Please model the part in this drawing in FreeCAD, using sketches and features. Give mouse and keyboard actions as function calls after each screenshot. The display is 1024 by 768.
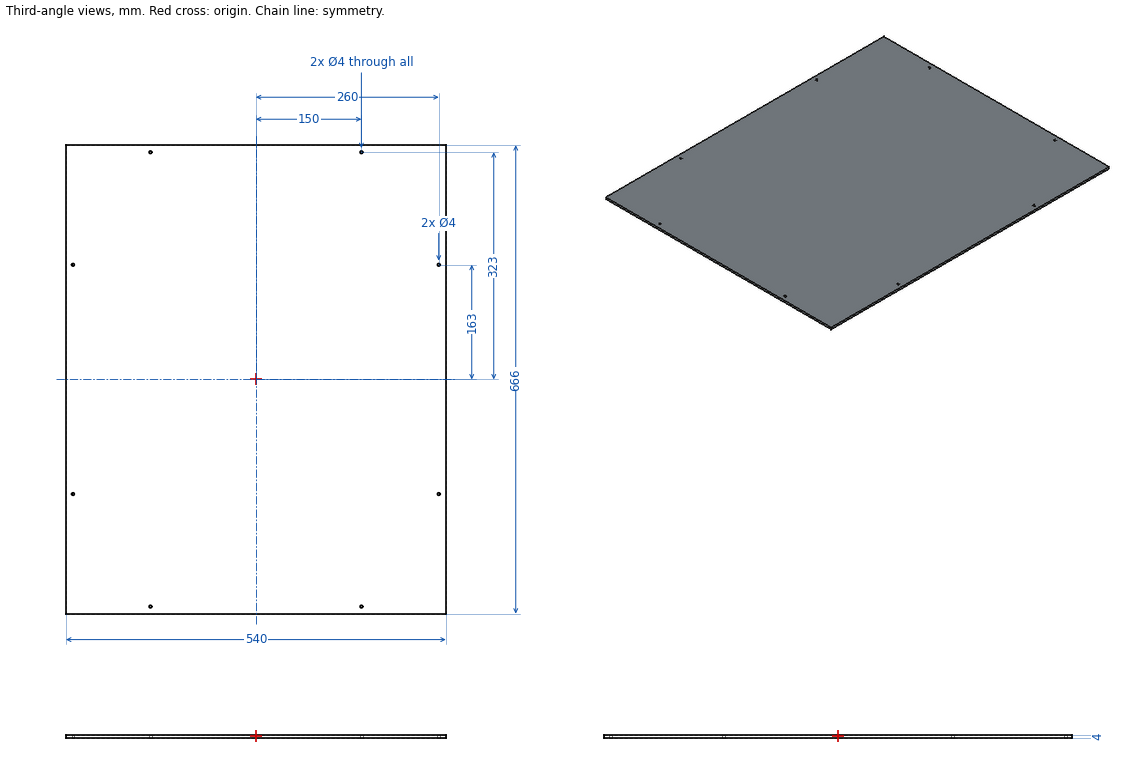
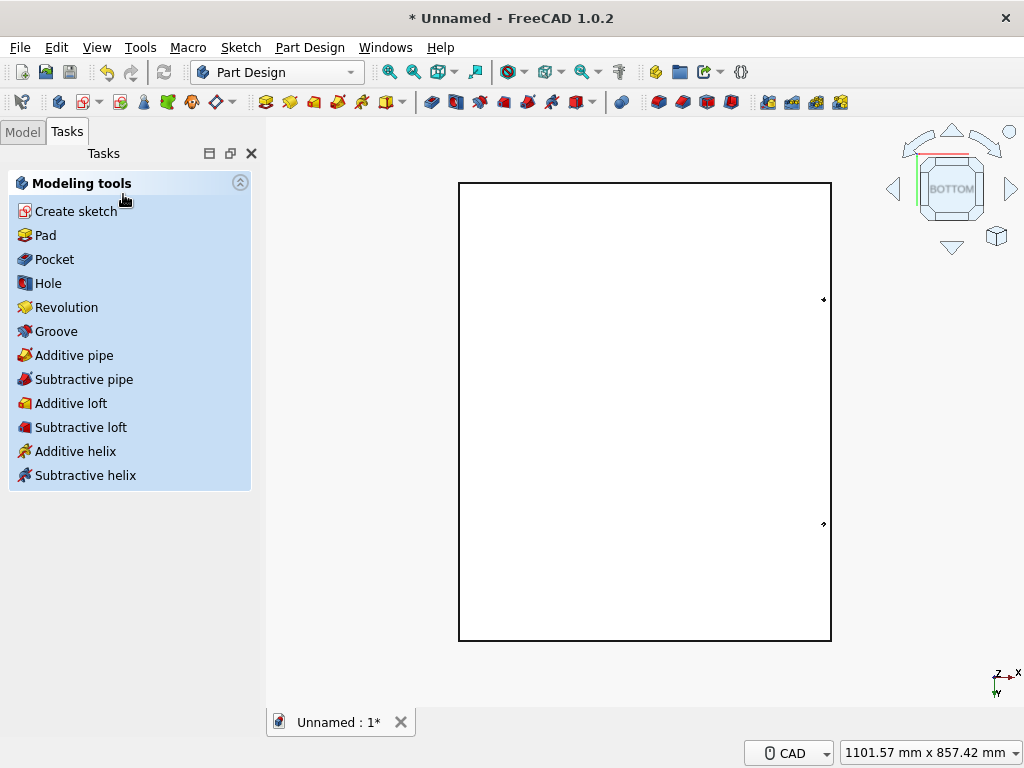
click(456, 102)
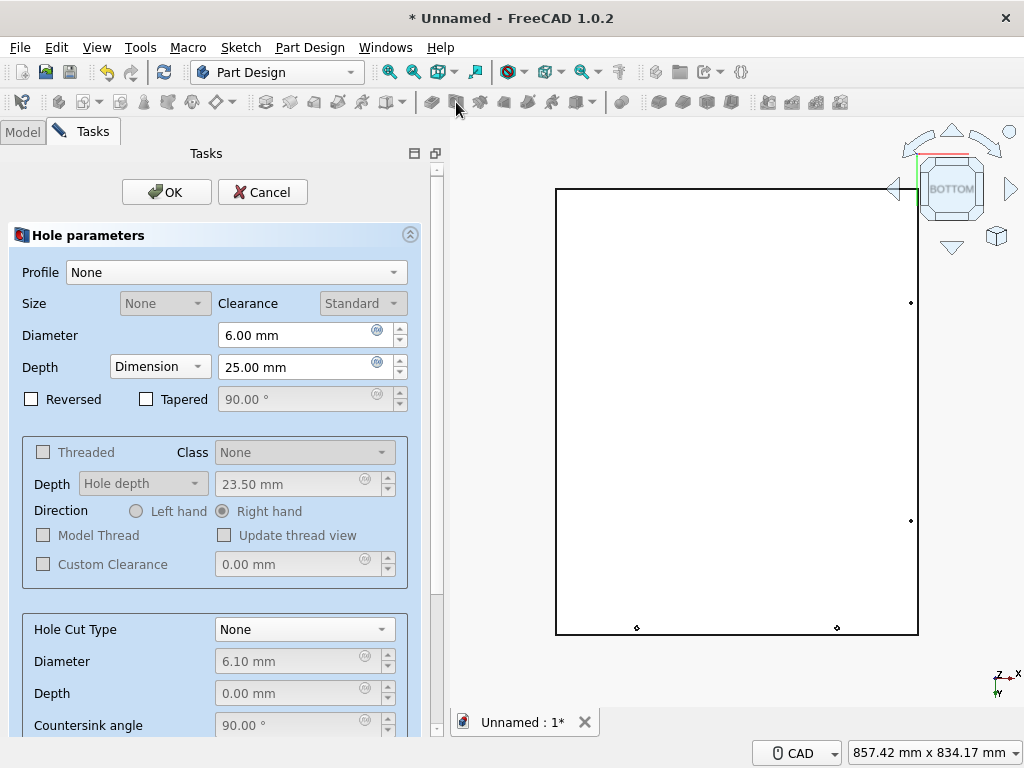
triple_click(305, 335)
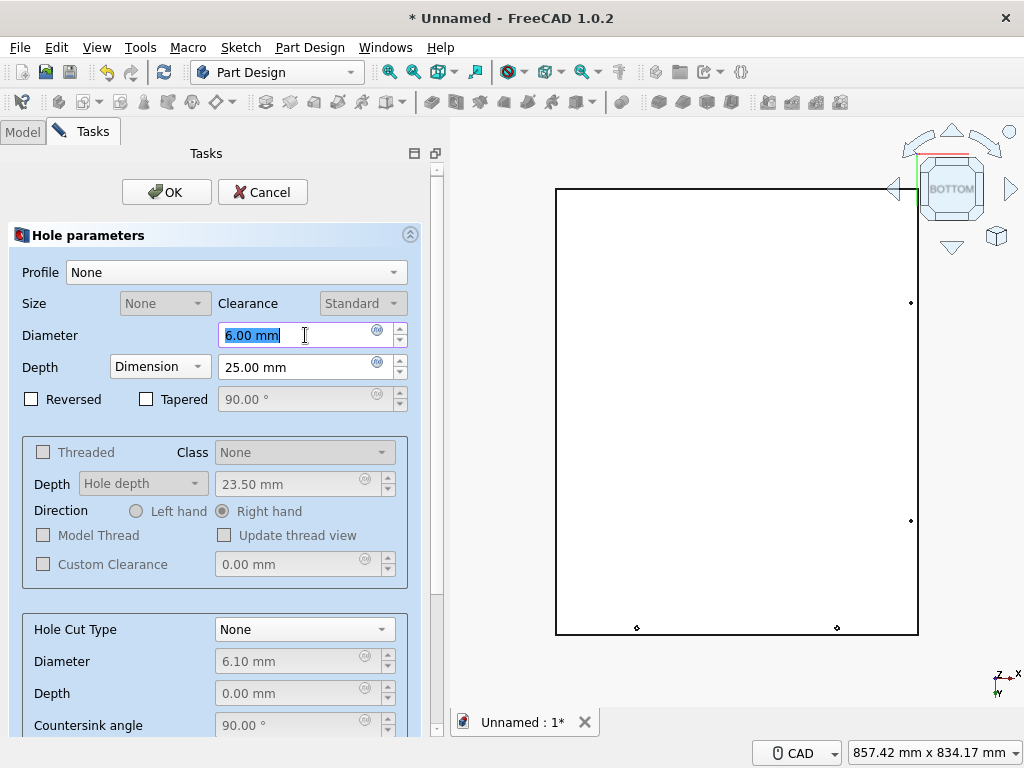
text(4)
key(Tab)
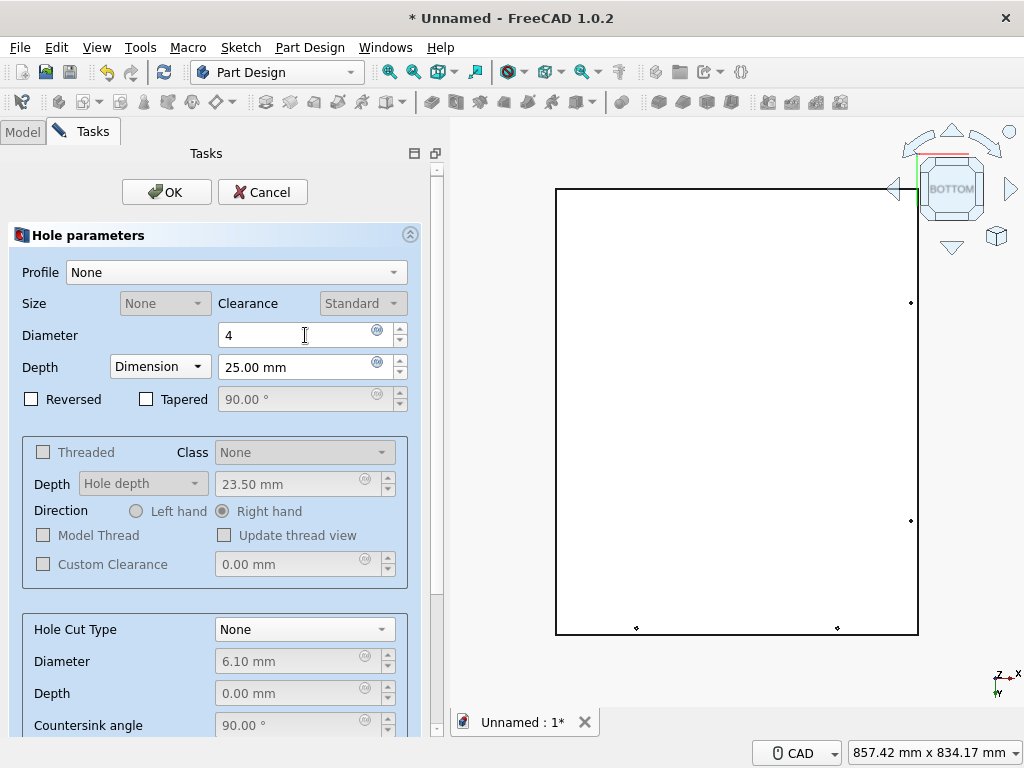
click(161, 366)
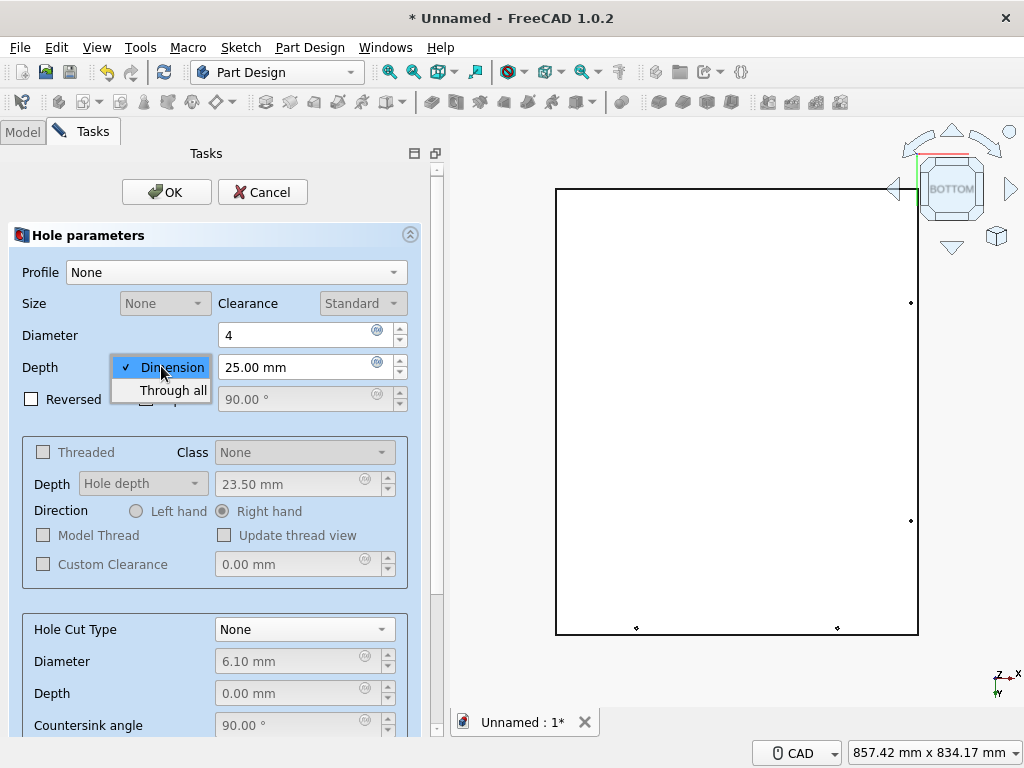
click(160, 390)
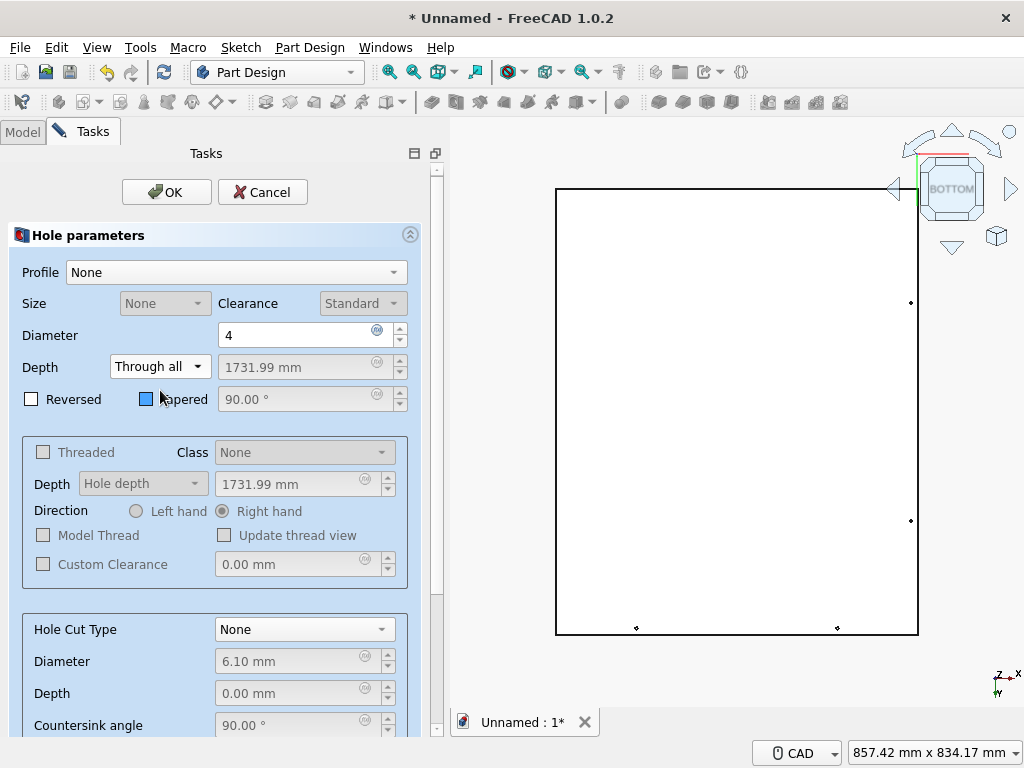
click(167, 192)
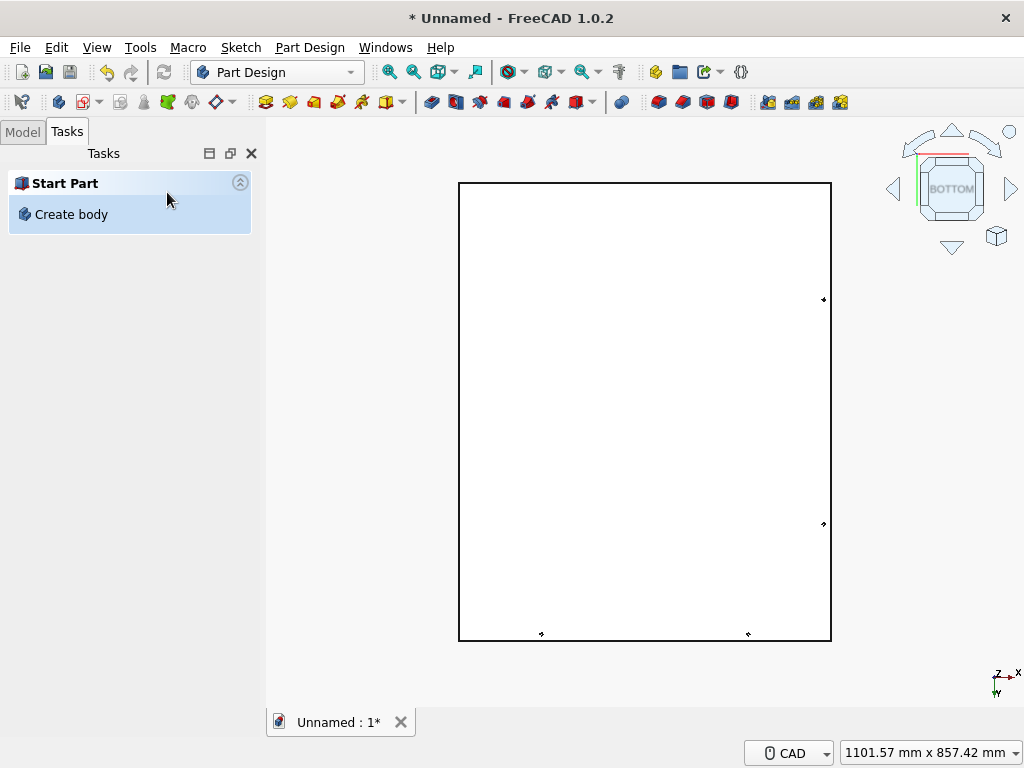
click(23, 131)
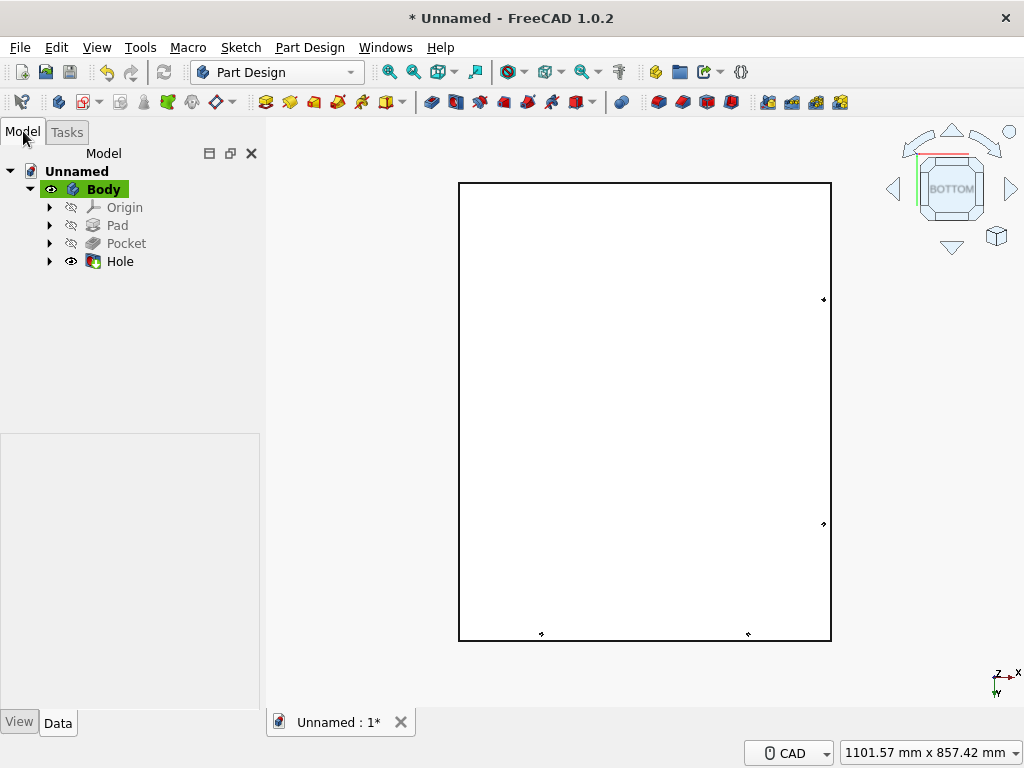
click(116, 261)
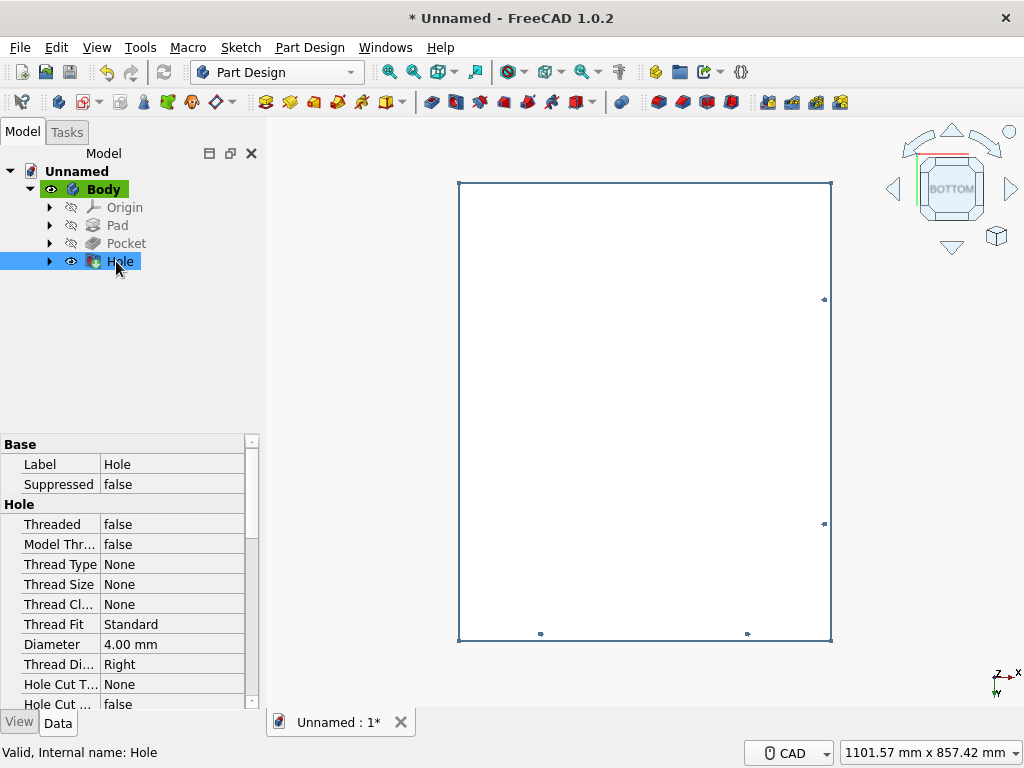
click(768, 102)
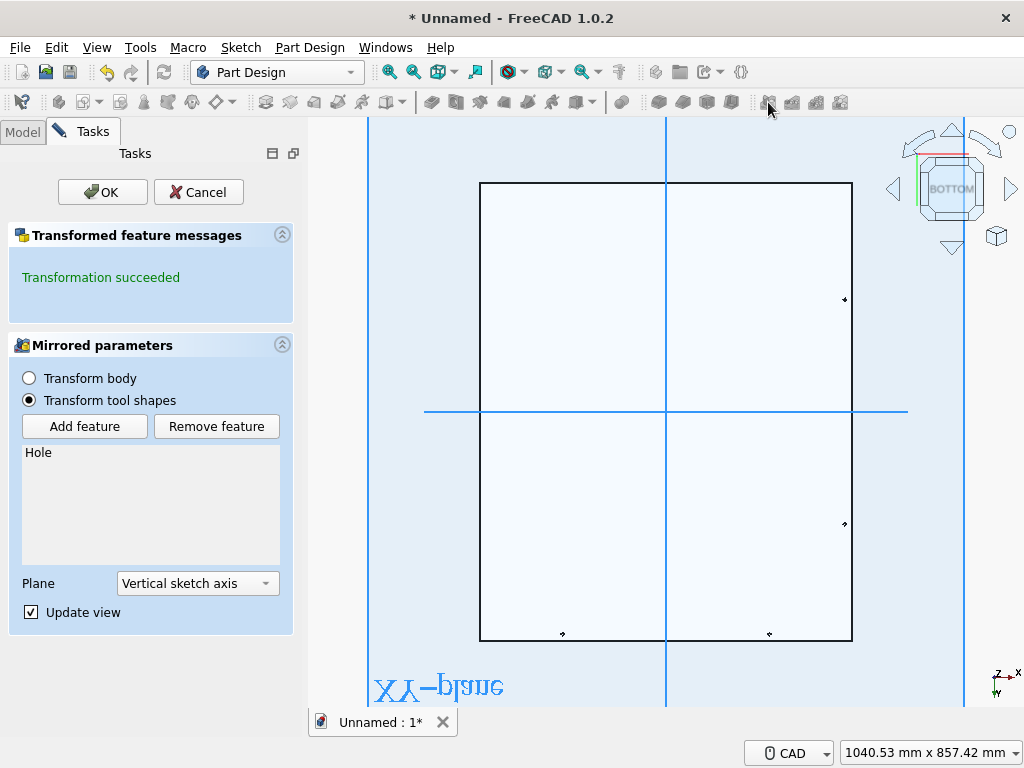
click(198, 584)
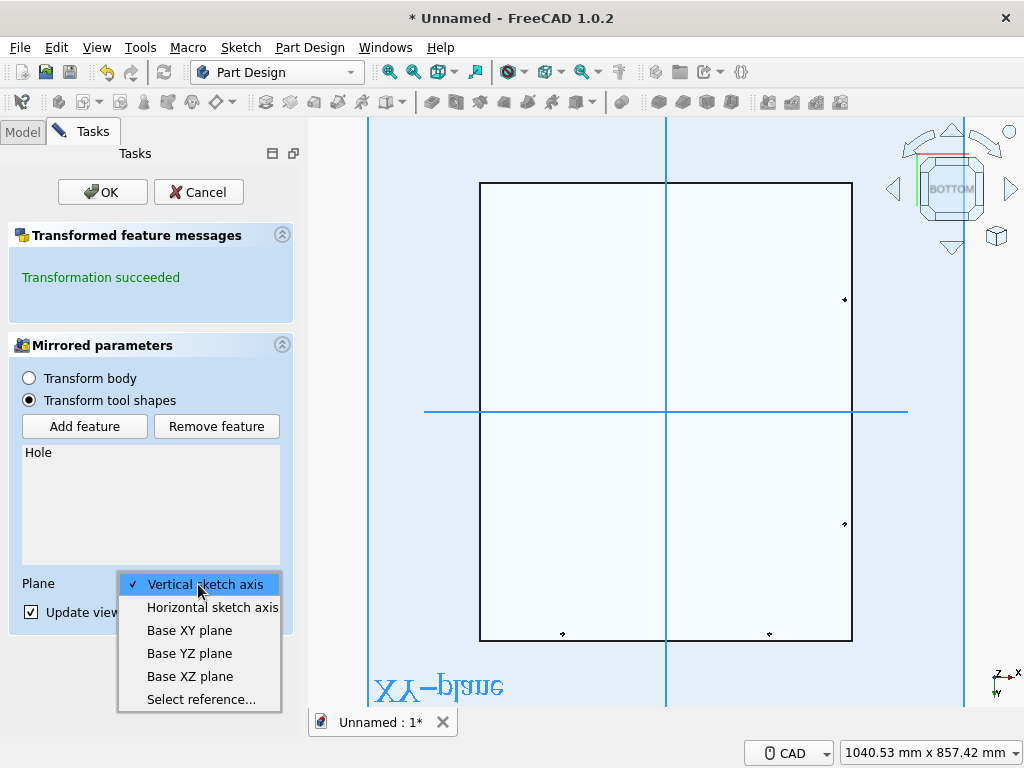
click(198, 676)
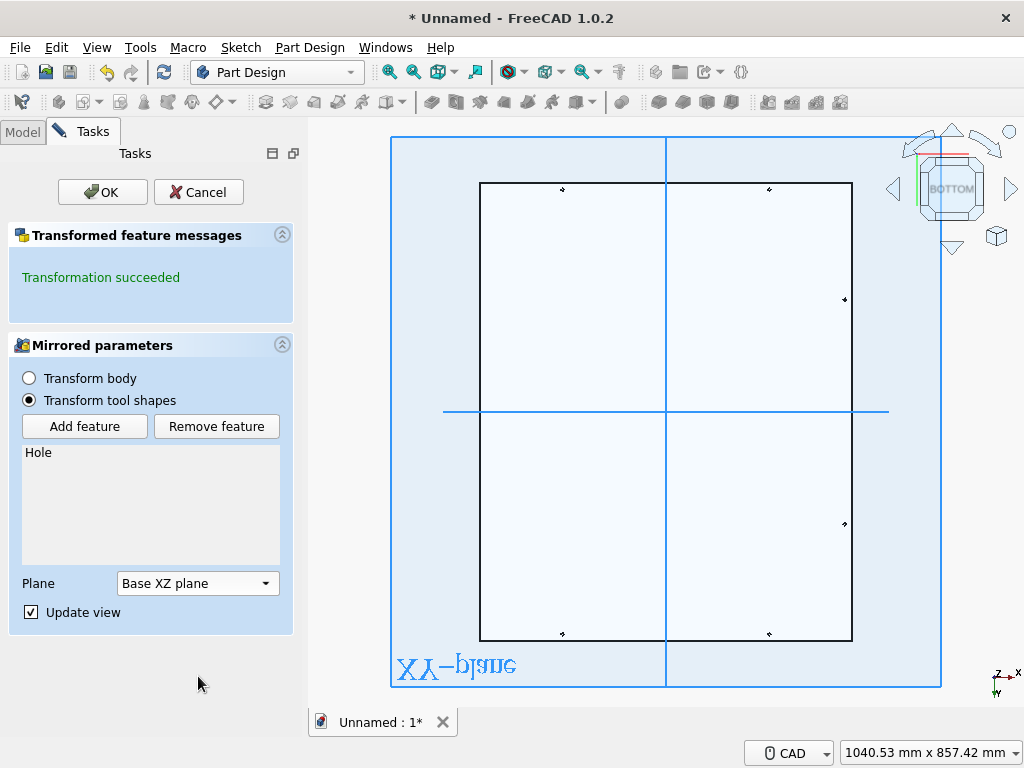
click(103, 192)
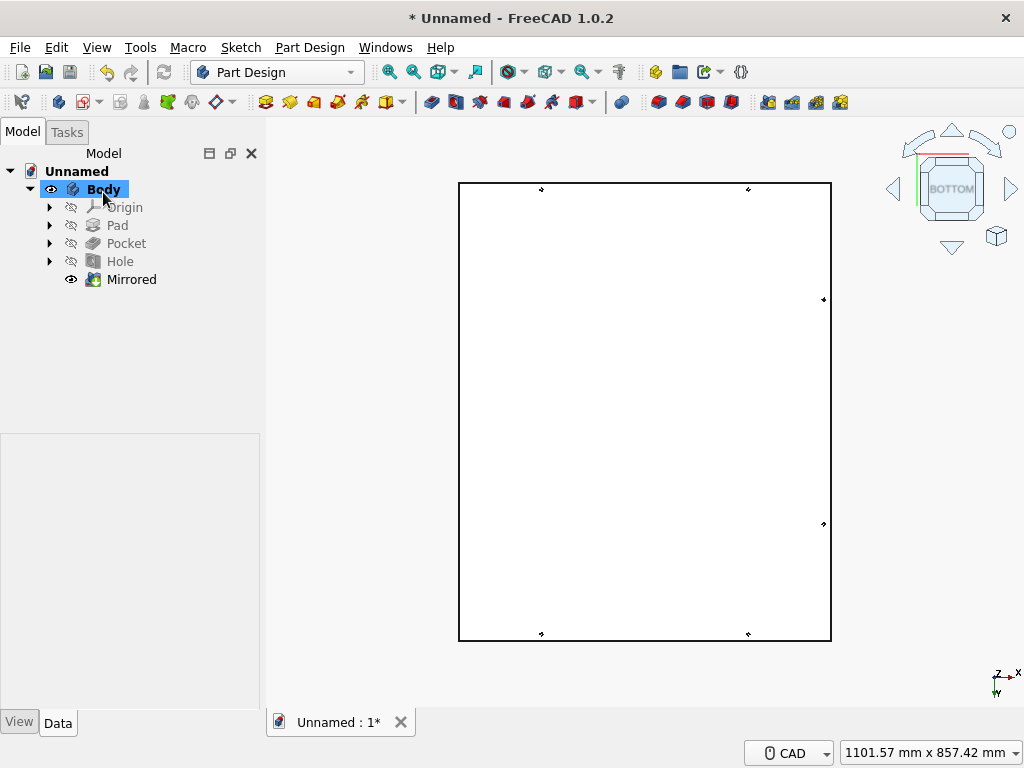
click(116, 243)